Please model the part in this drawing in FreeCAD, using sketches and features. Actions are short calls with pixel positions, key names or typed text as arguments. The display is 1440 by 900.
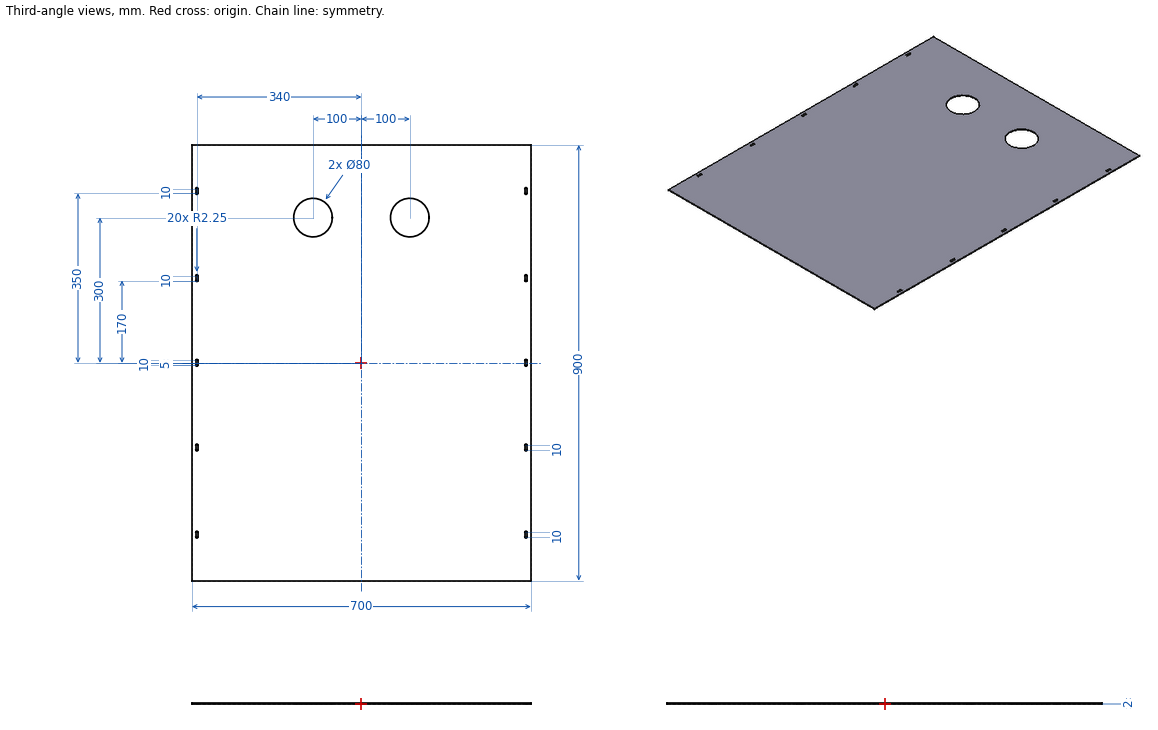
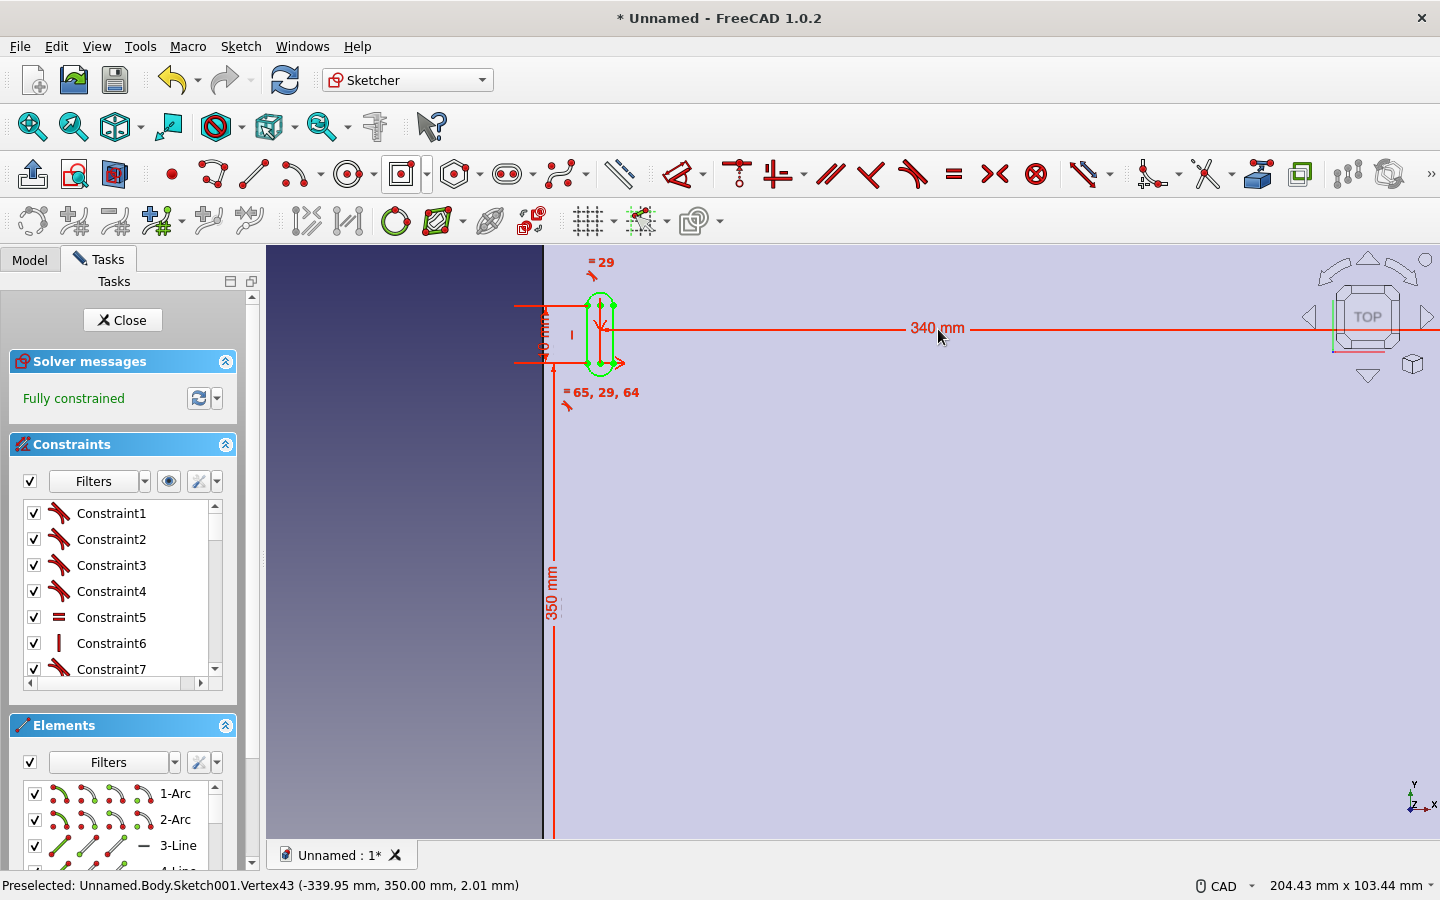
click(123, 320)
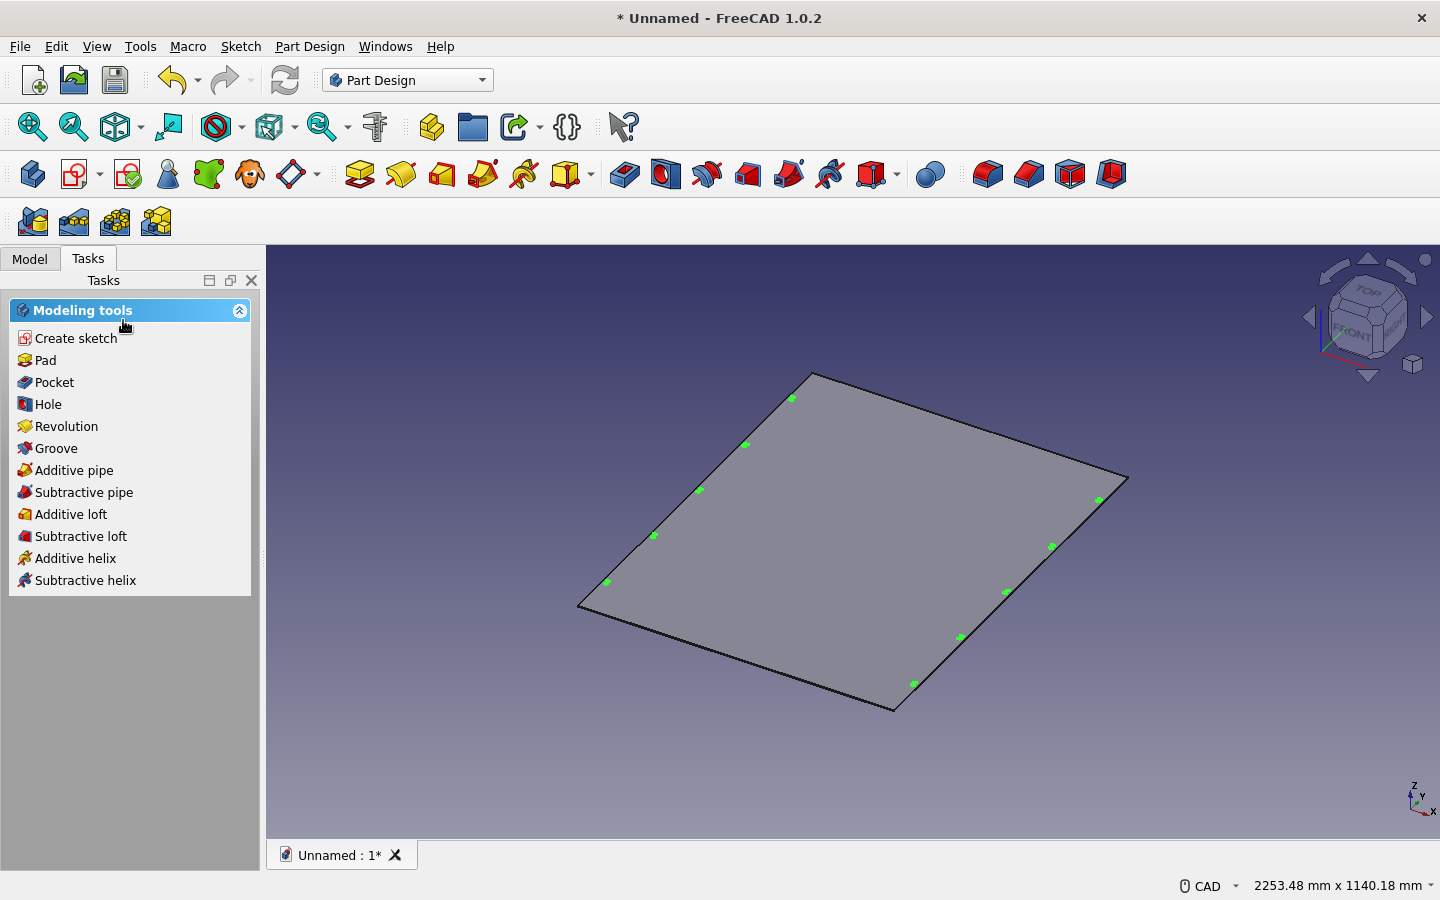
click(625, 174)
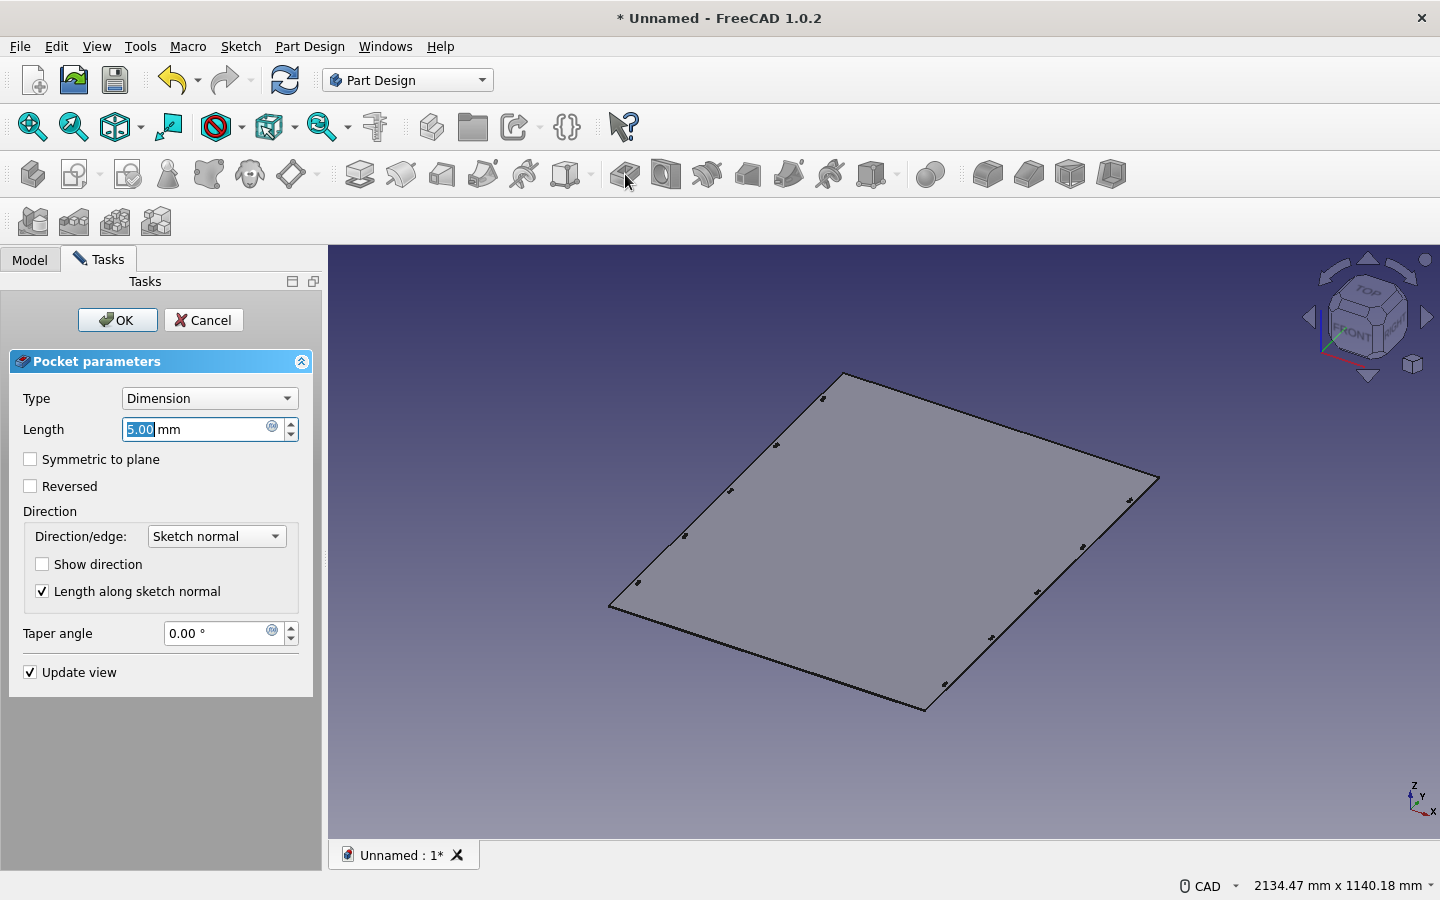
text(10)
key(Tab)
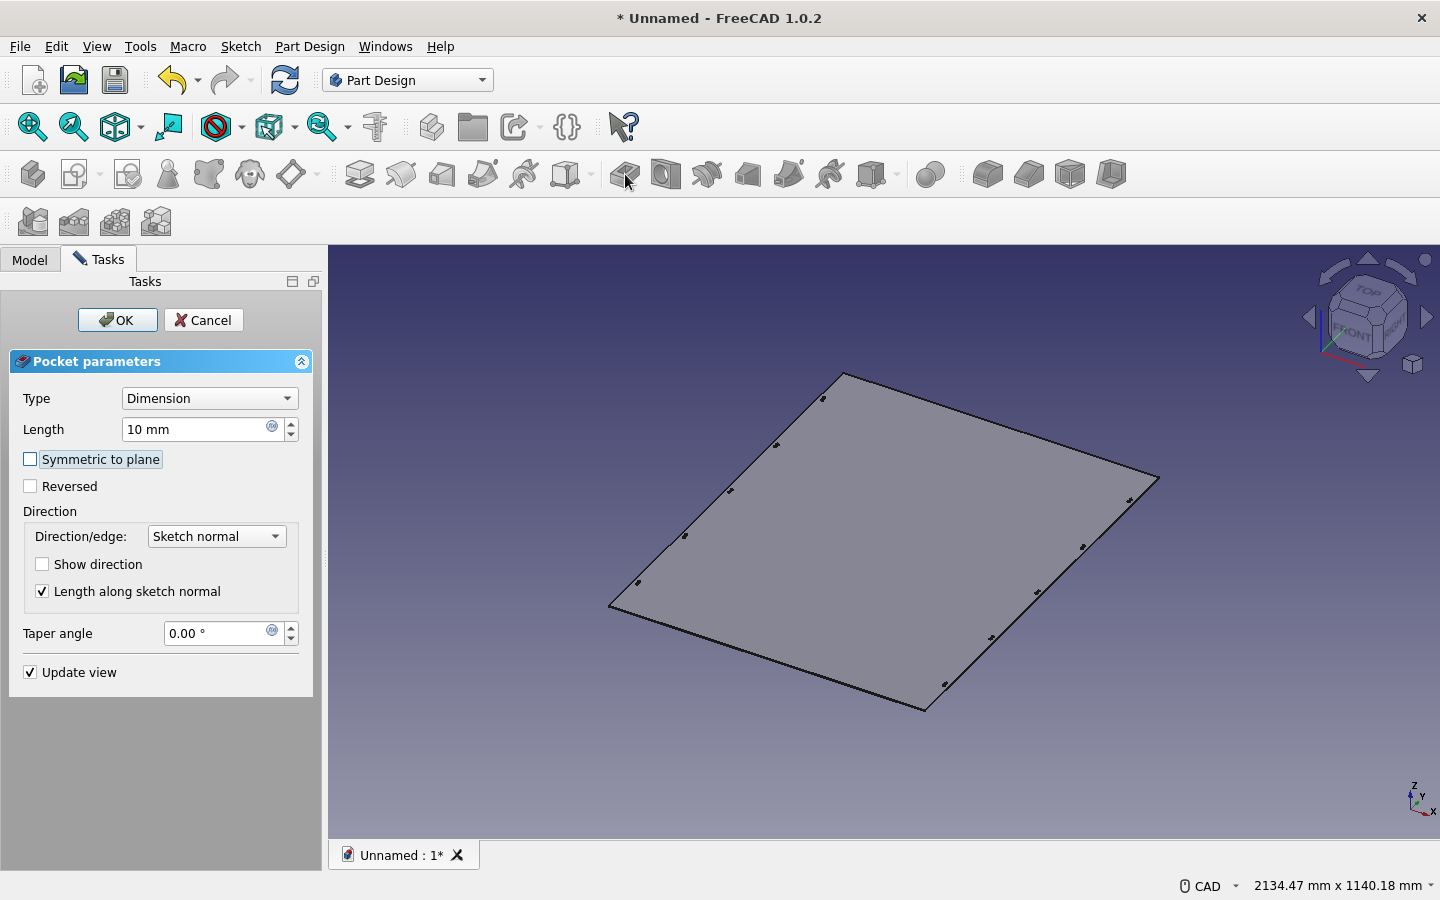
click(118, 320)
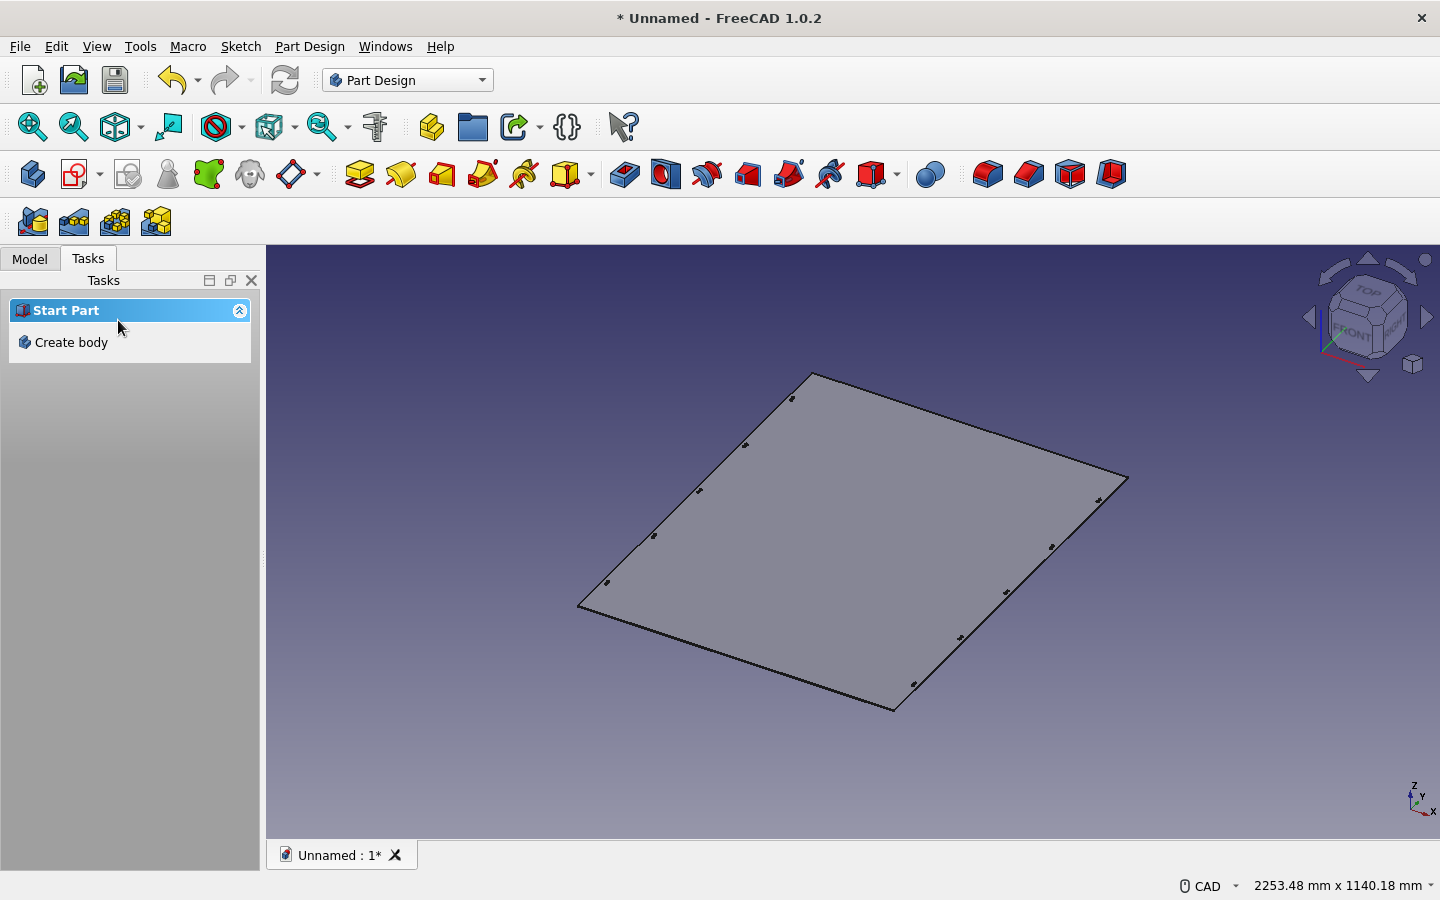
click(853, 541)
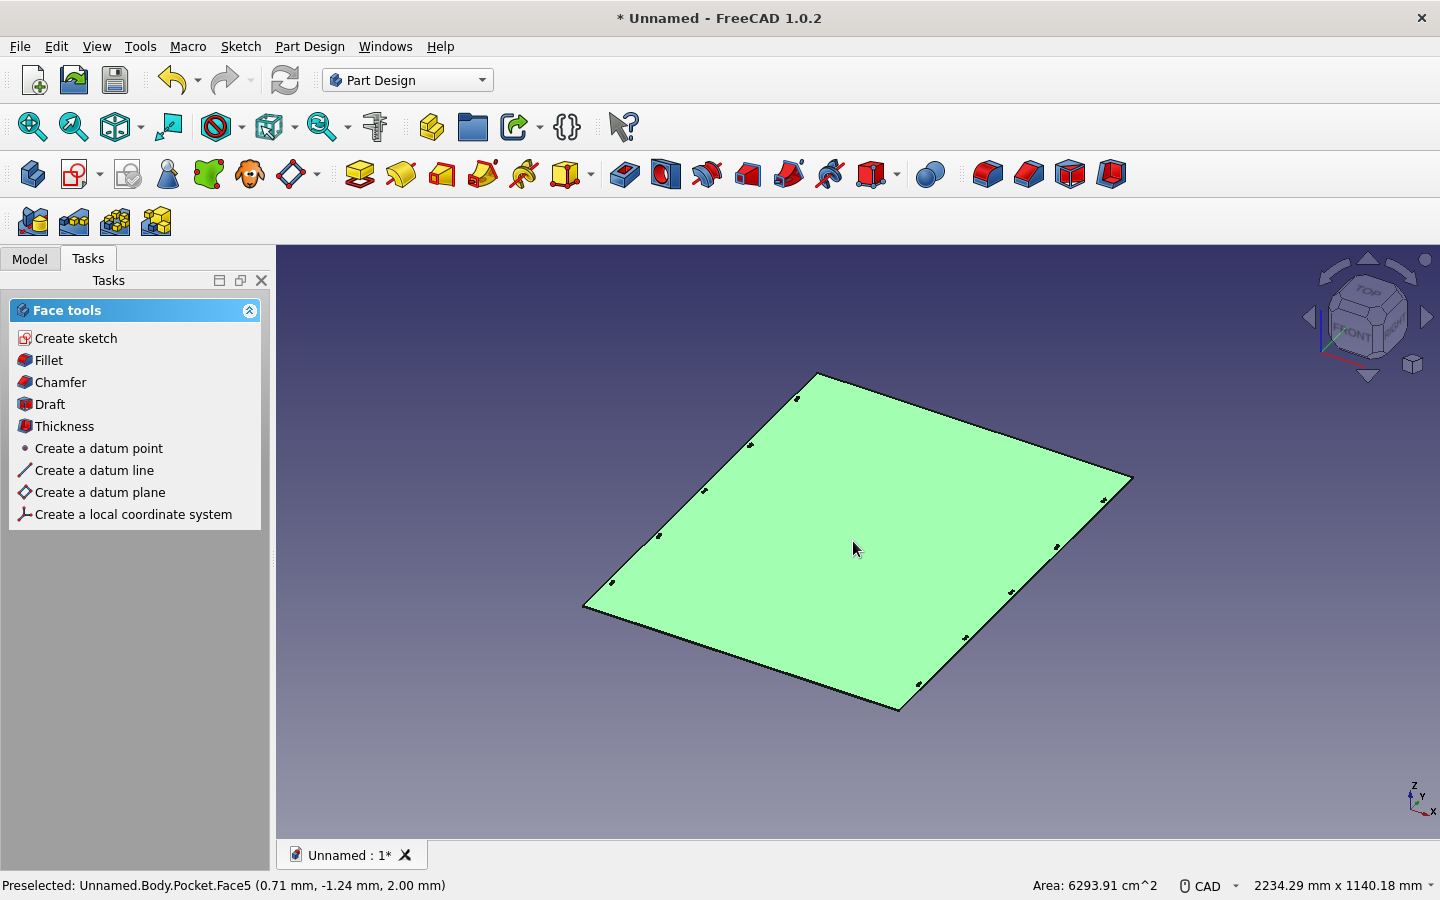
click(74, 174)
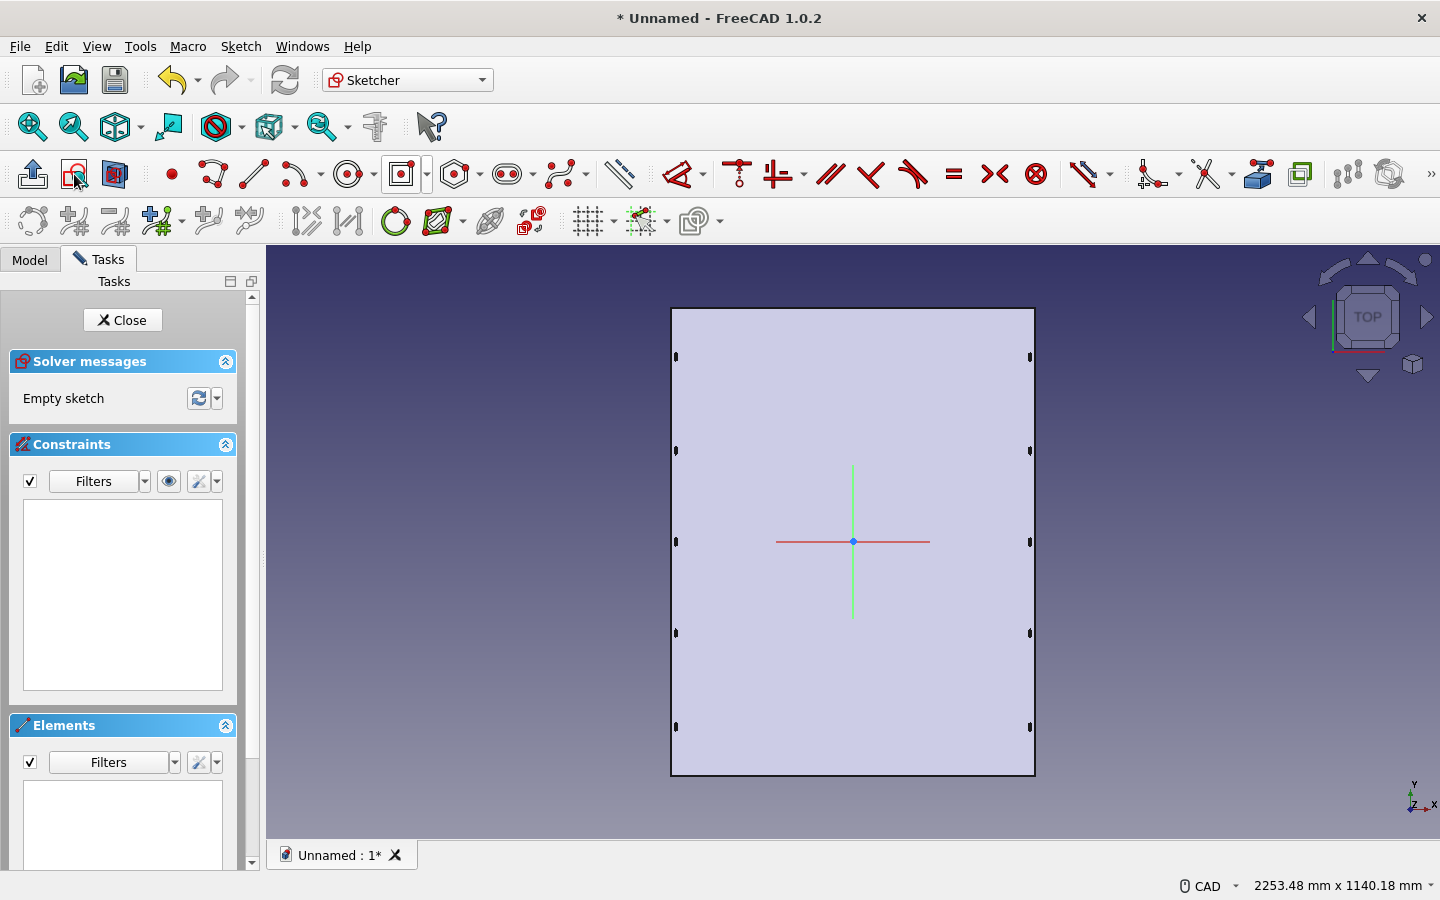
scroll(909, 381, up, 4)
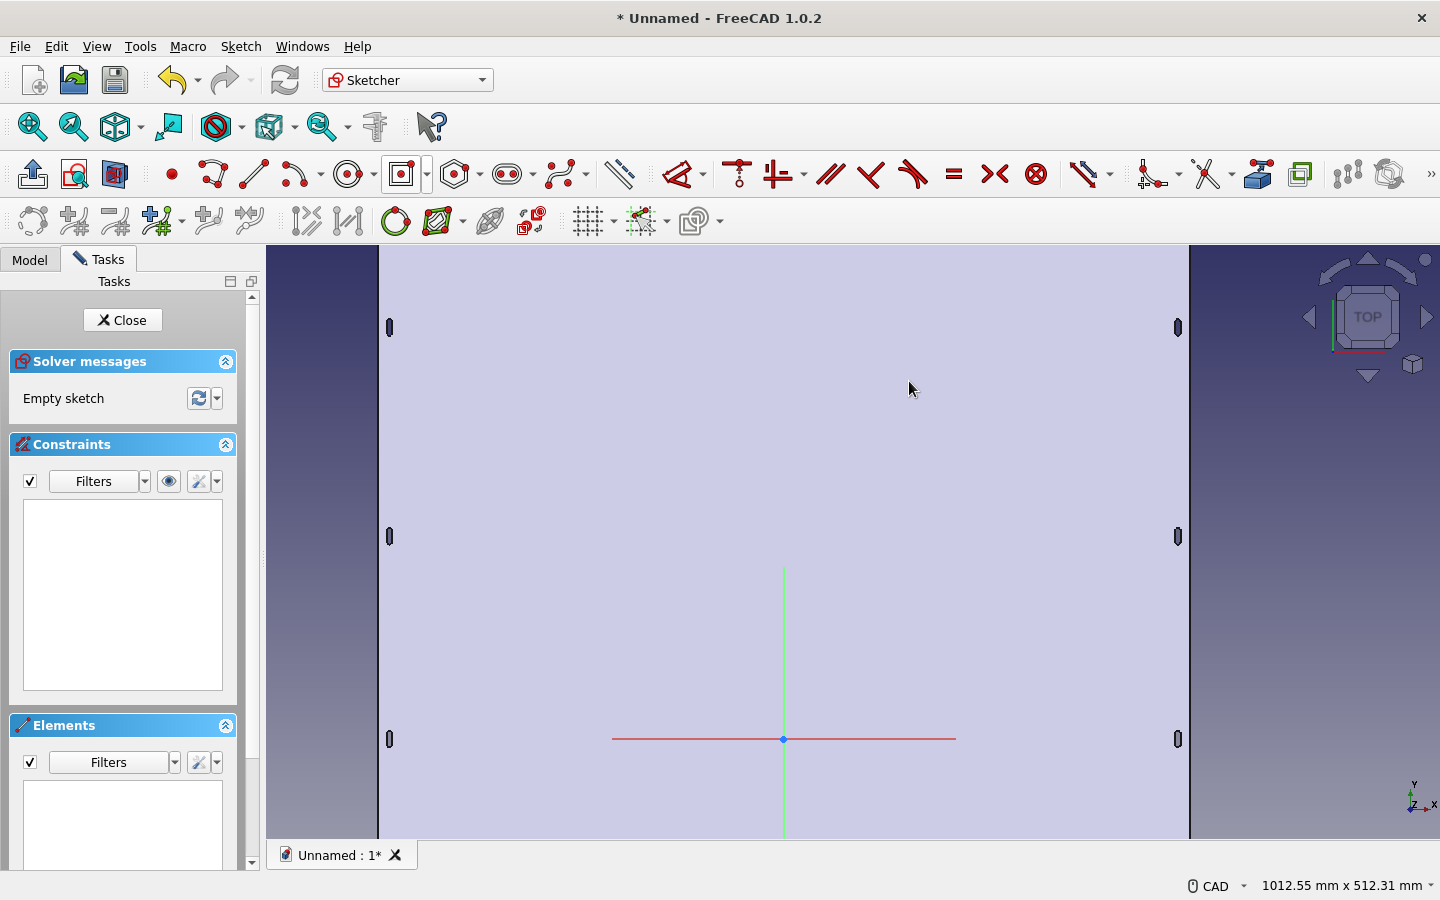
key(g)
key(c)